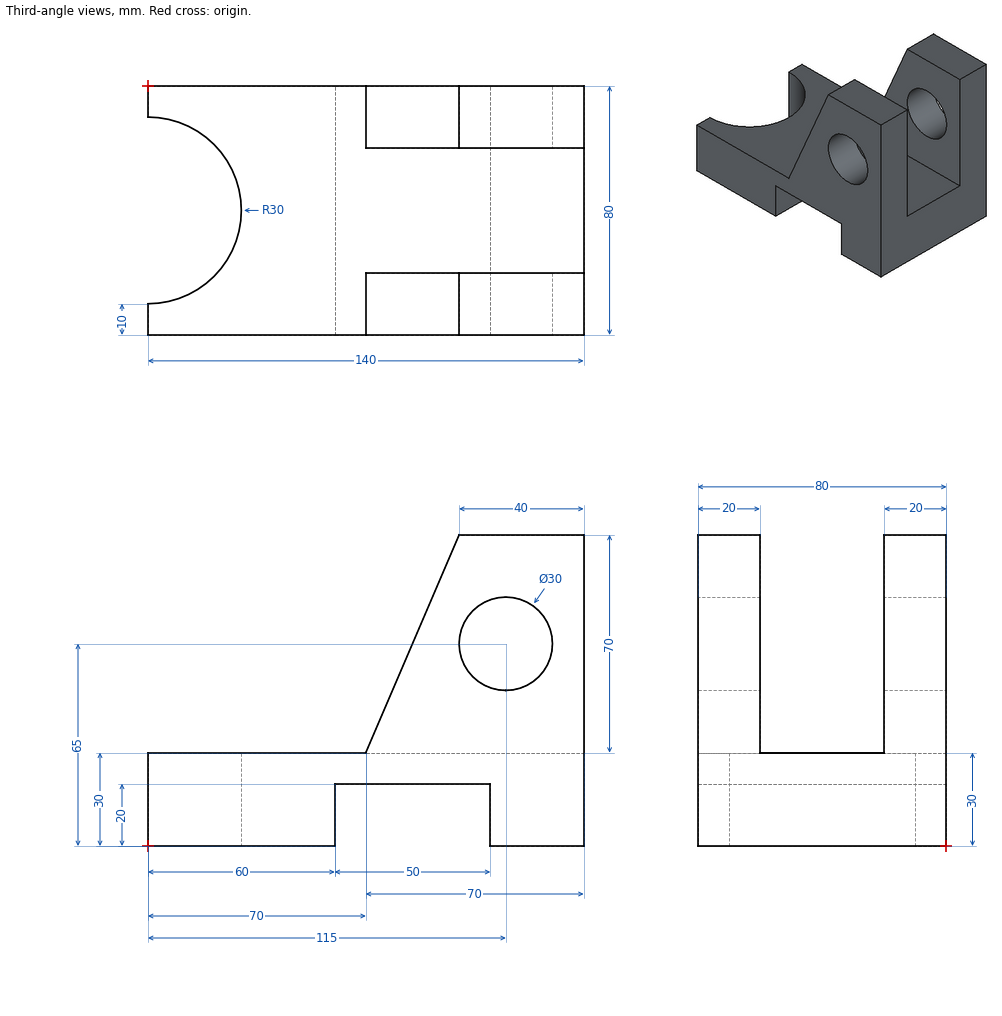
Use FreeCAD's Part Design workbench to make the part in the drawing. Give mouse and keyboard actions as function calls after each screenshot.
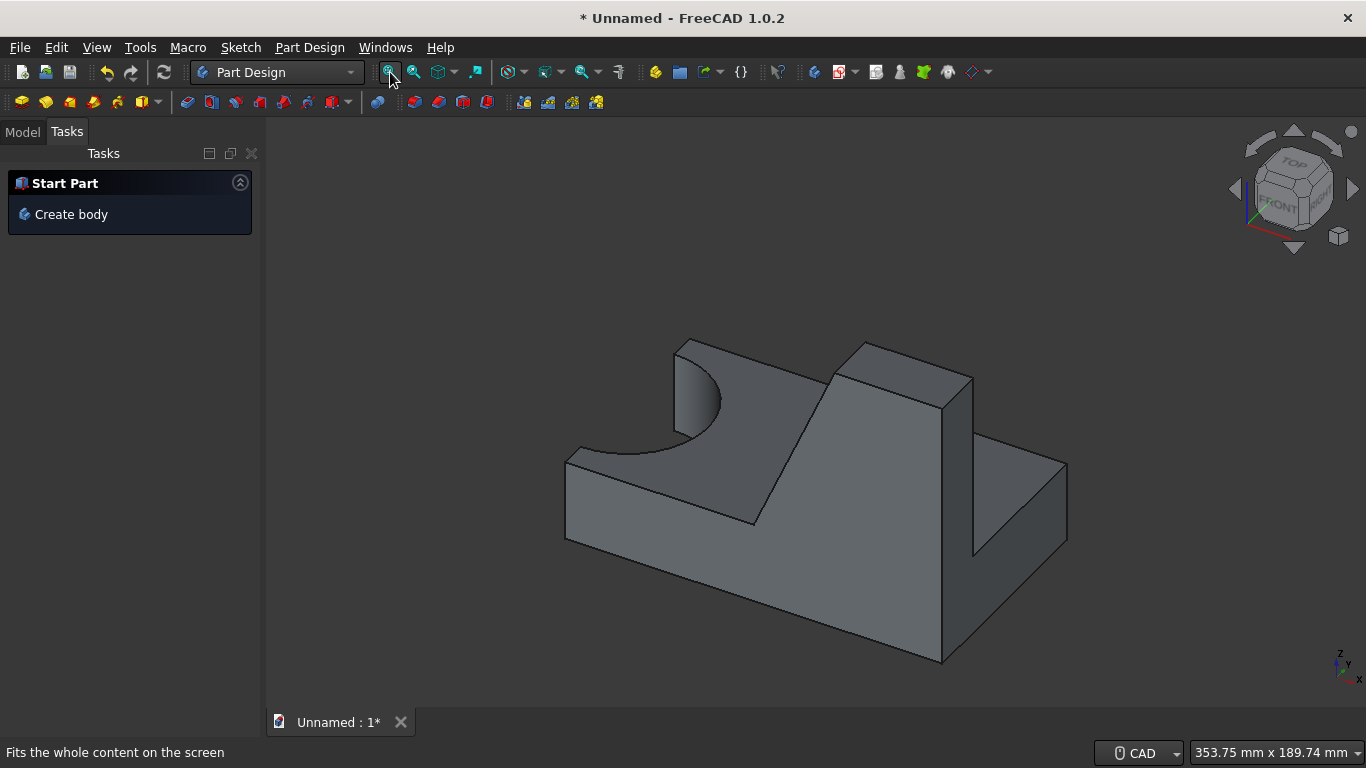
key(4)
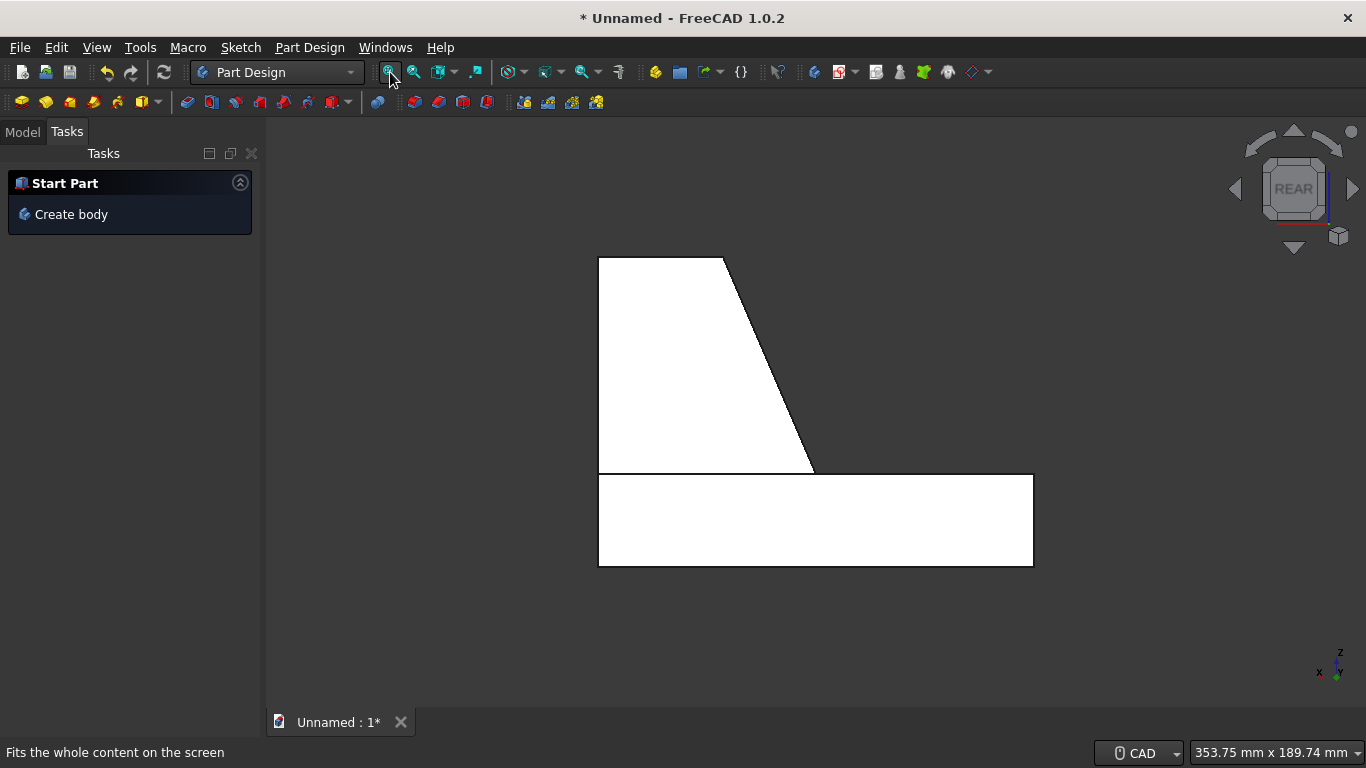
click(692, 520)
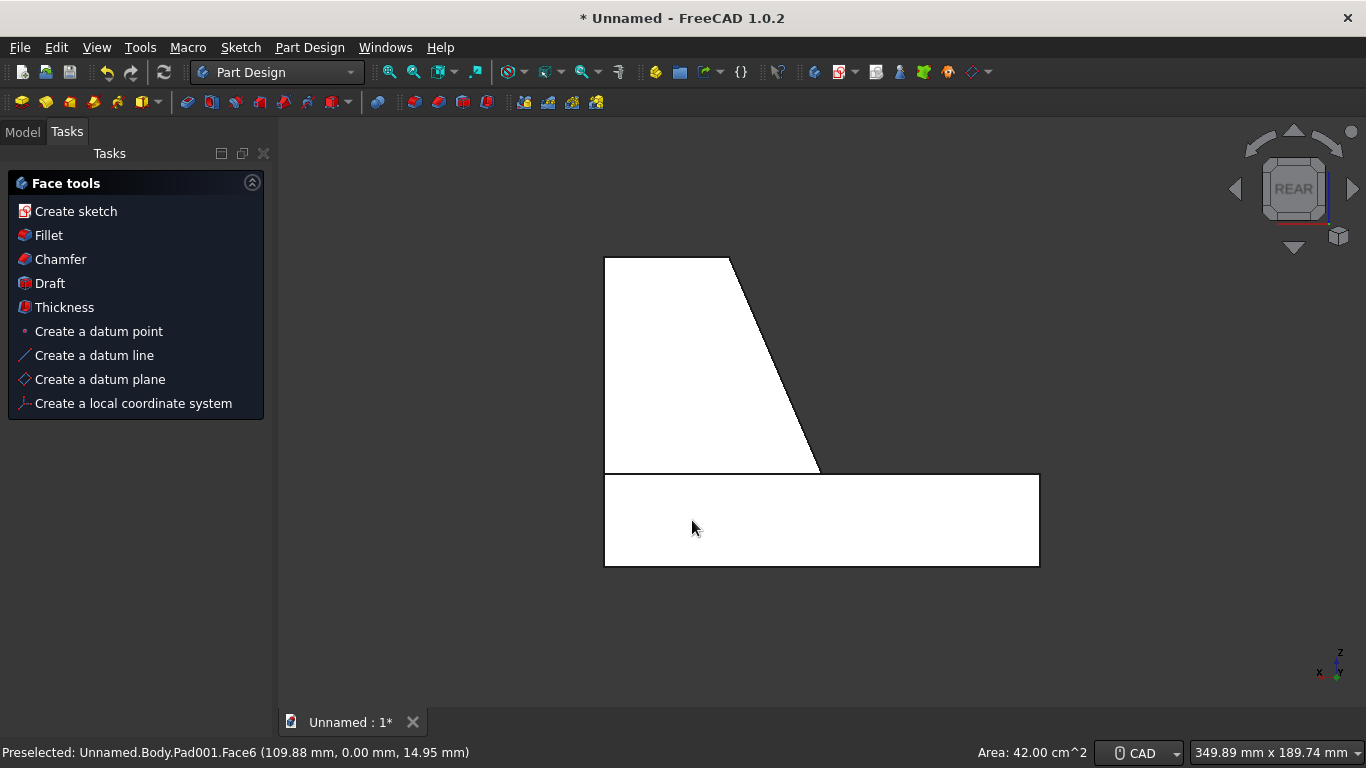
click(840, 72)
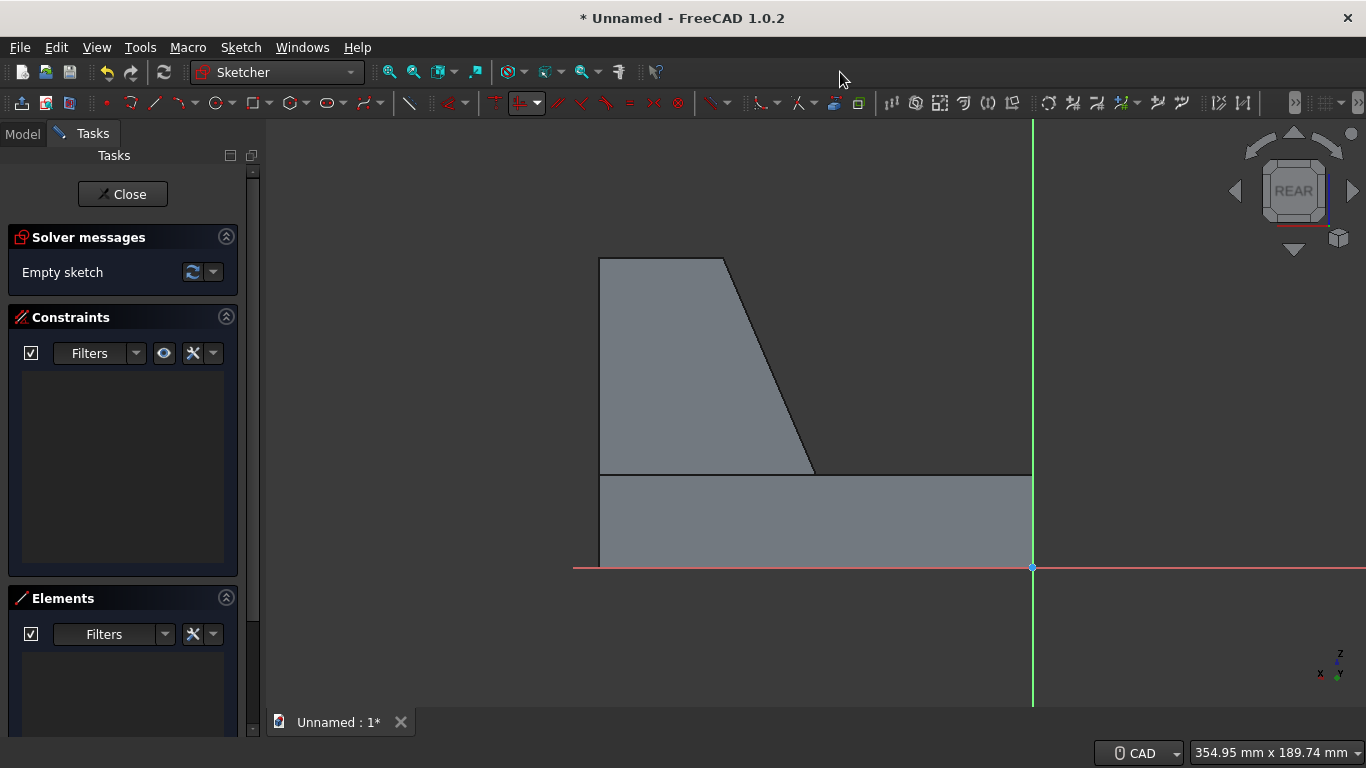
click(132, 104)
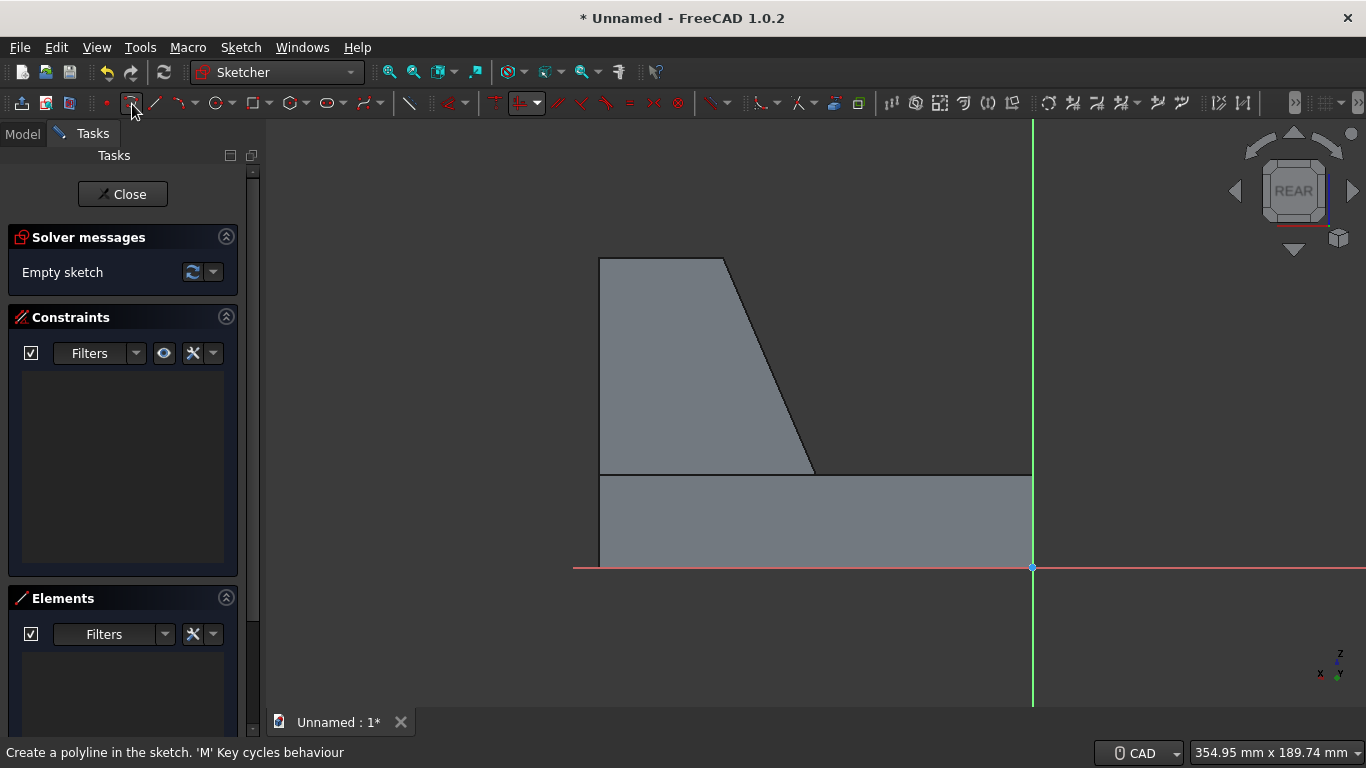
click(816, 475)
click(723, 258)
click(599, 258)
click(599, 475)
click(816, 476)
key(Escape)
key(Escape)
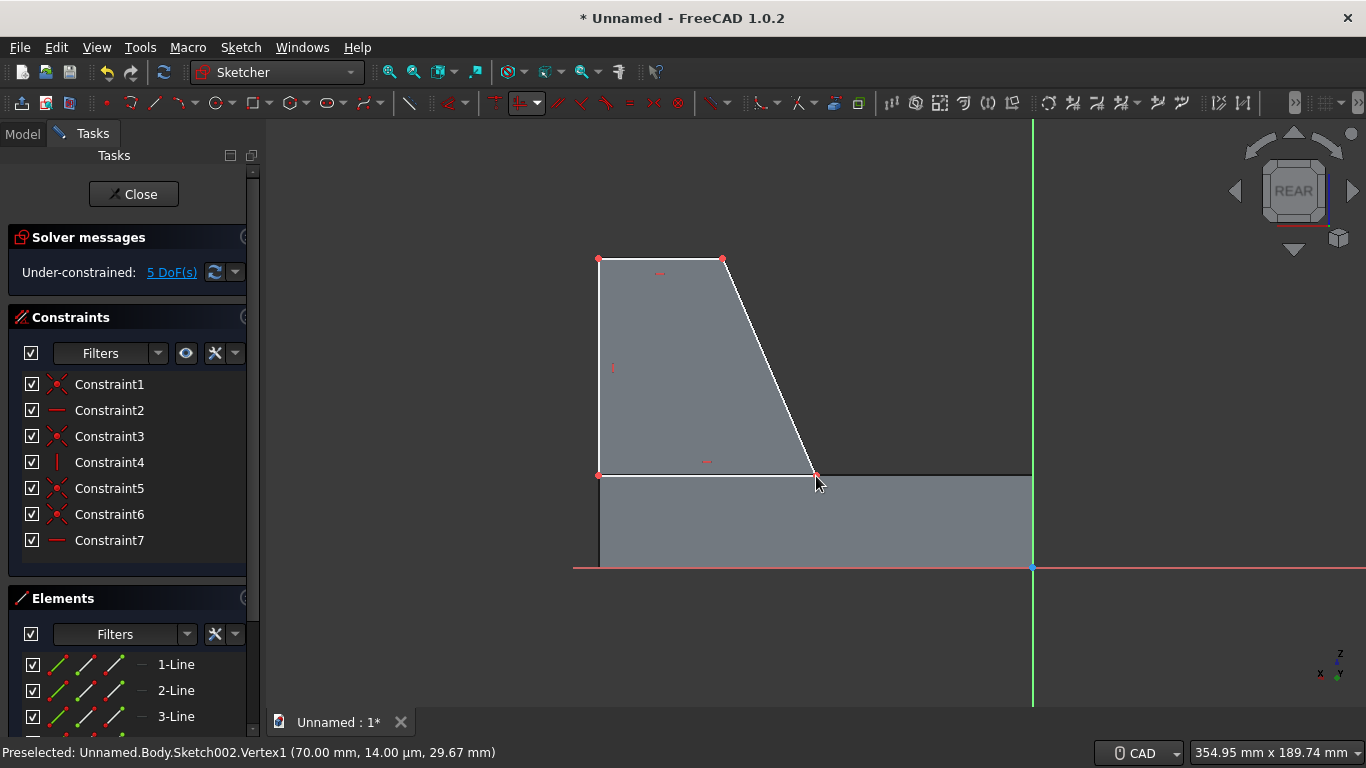
click(448, 104)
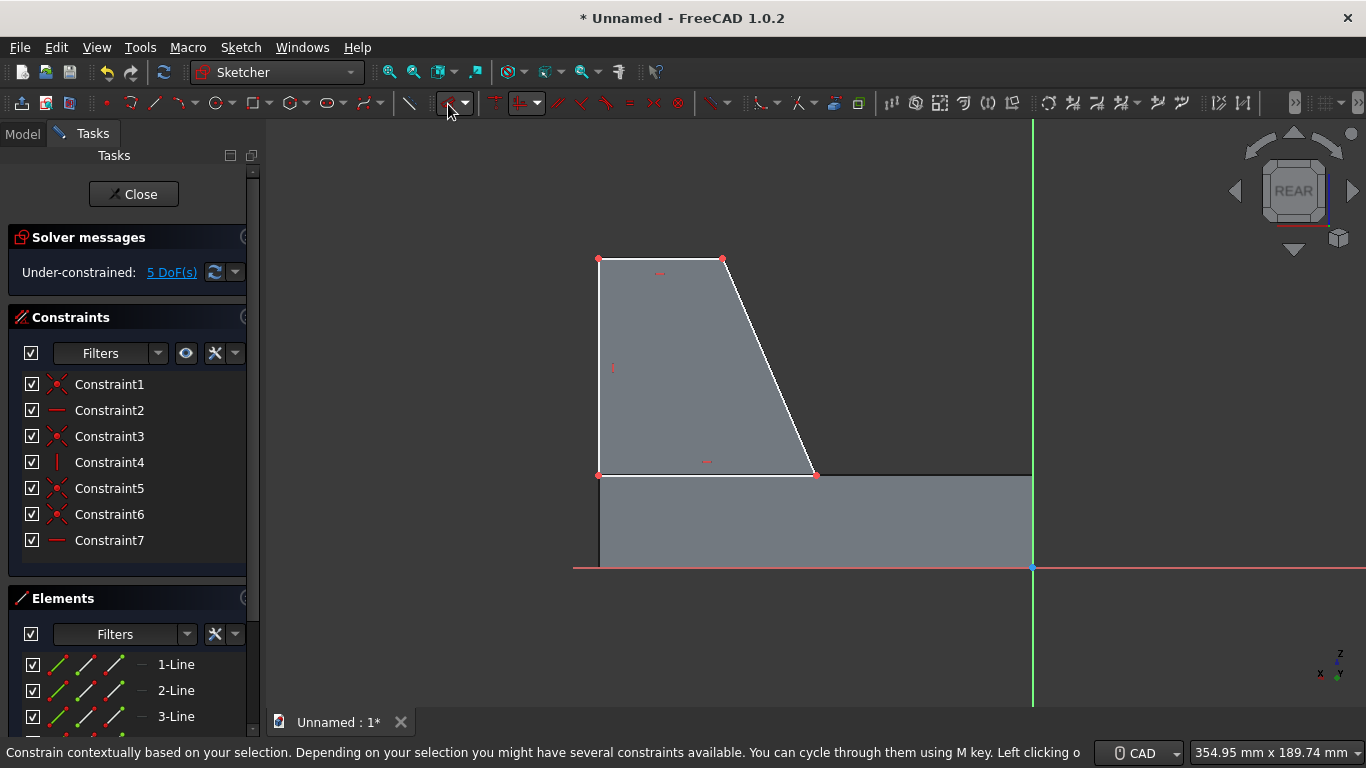
click(686, 259)
click(661, 225)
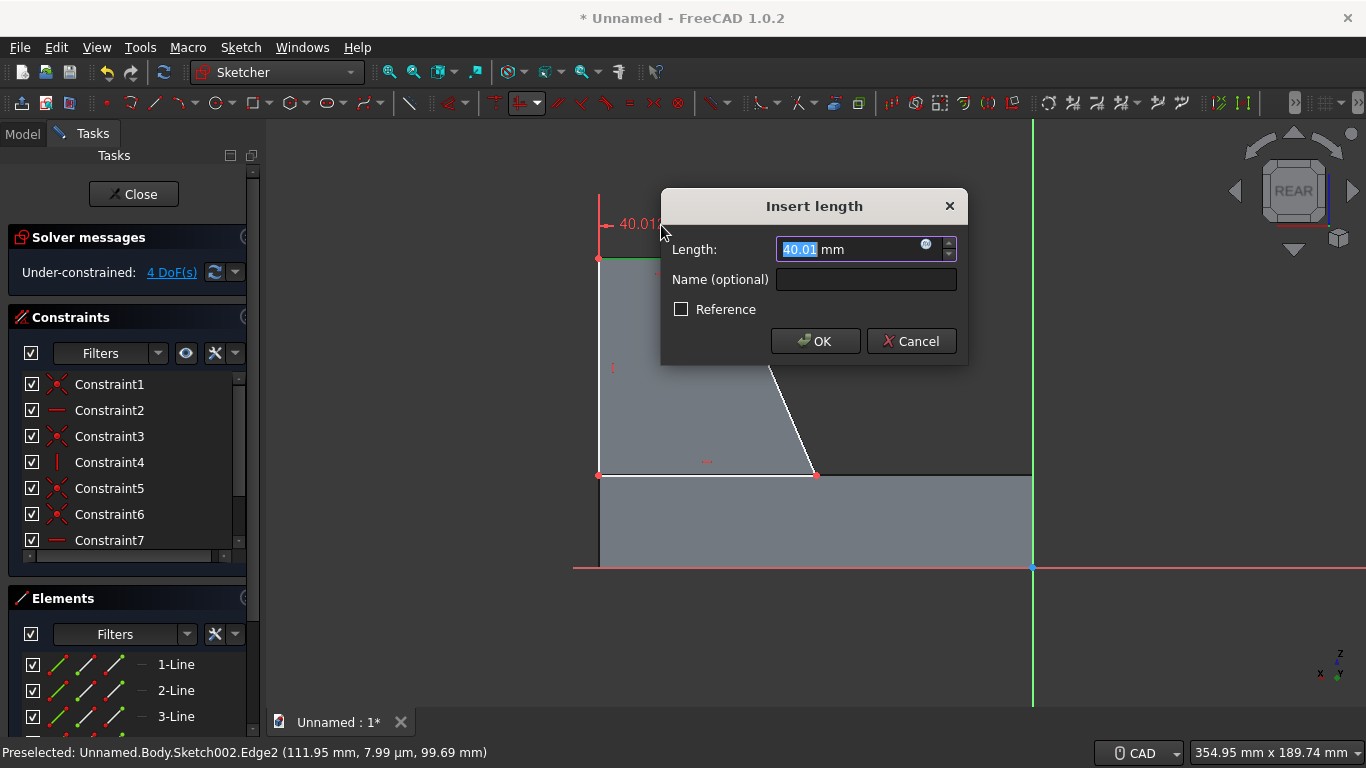
text(40)
key(Return)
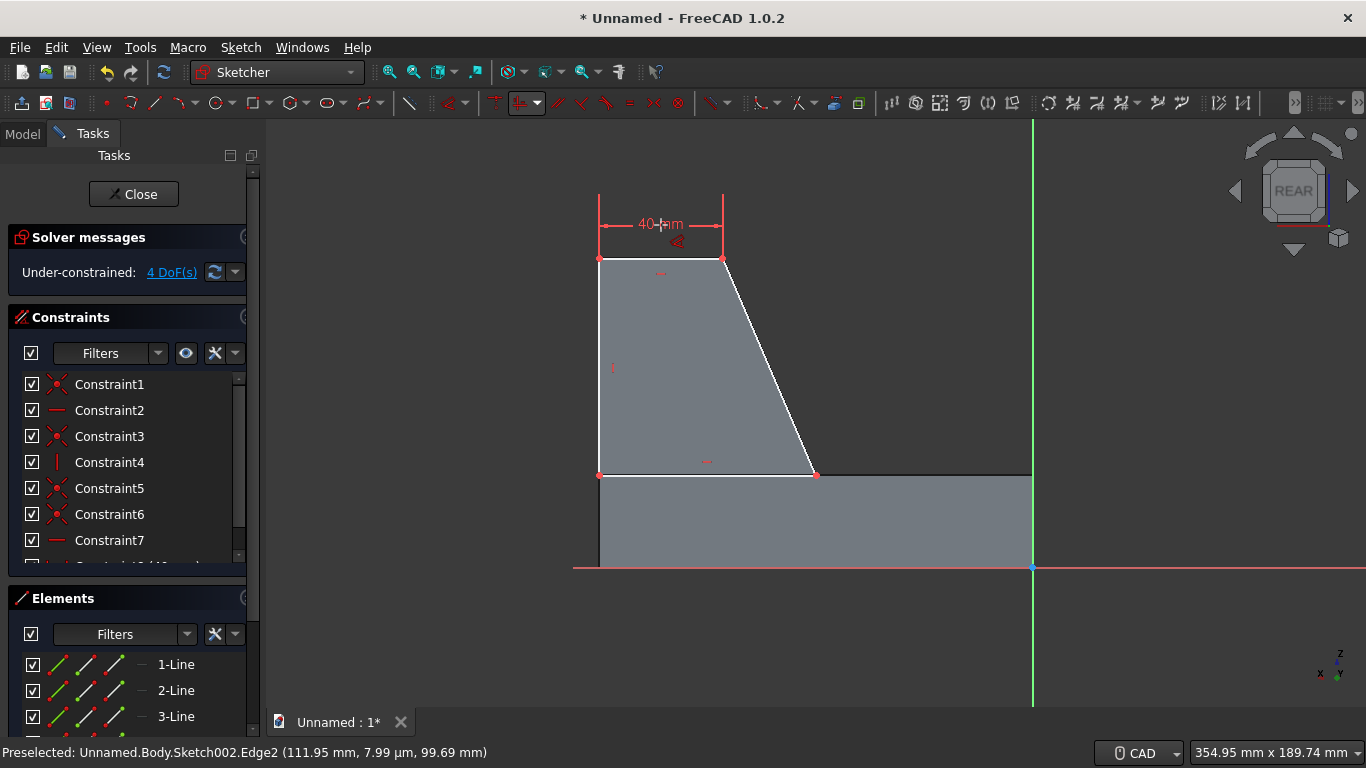
click(599, 324)
click(565, 367)